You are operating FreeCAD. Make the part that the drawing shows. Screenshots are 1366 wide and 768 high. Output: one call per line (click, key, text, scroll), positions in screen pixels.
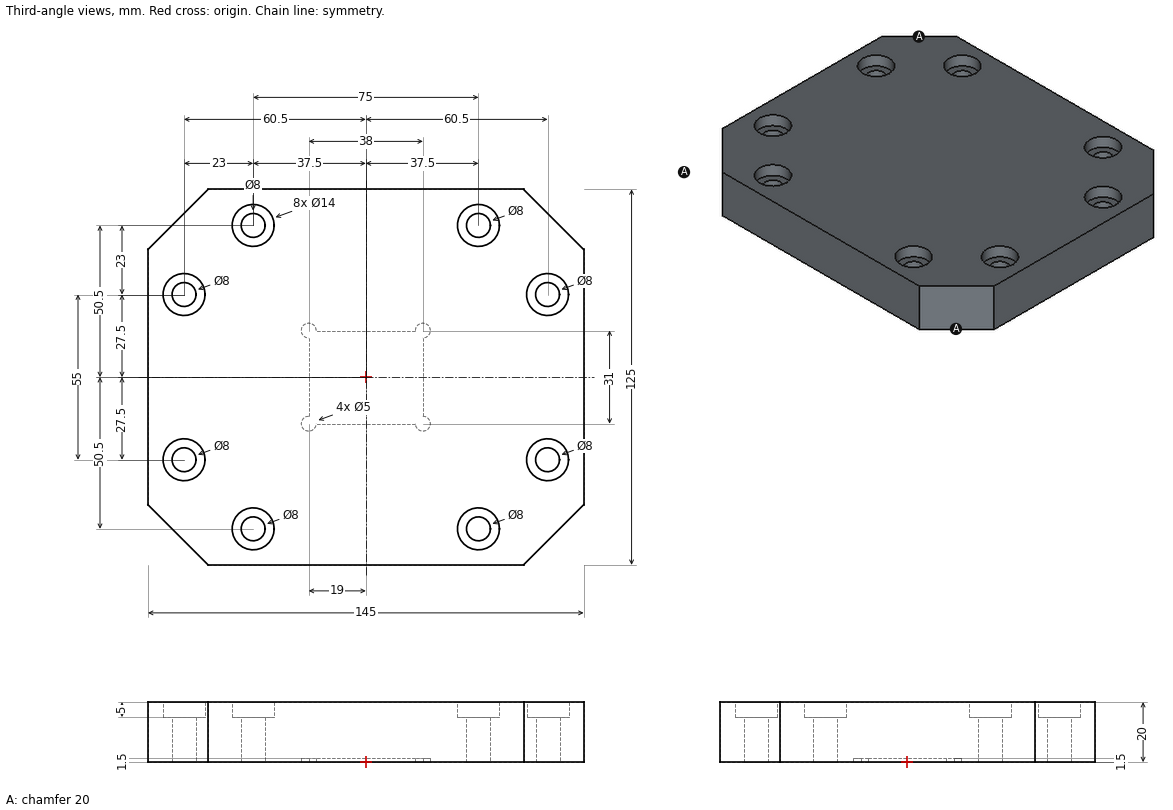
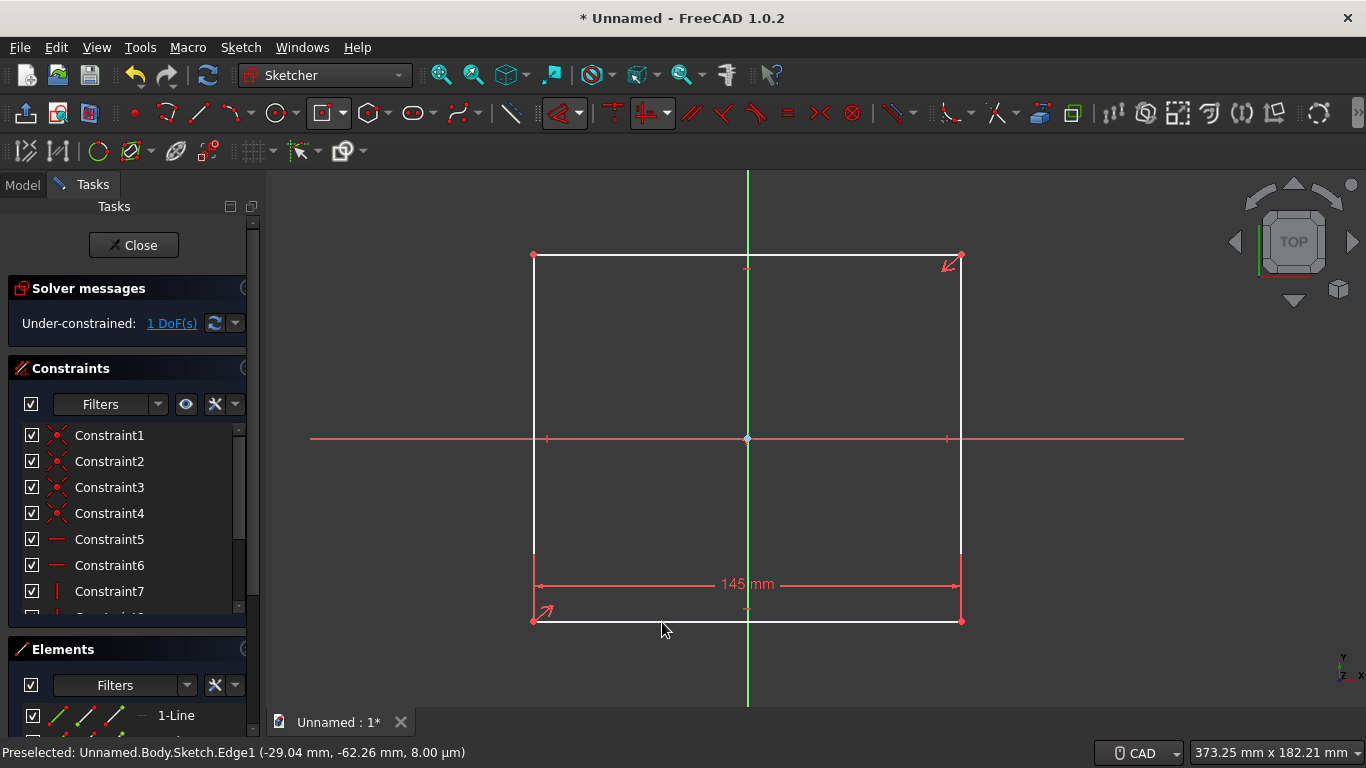
click(961, 512)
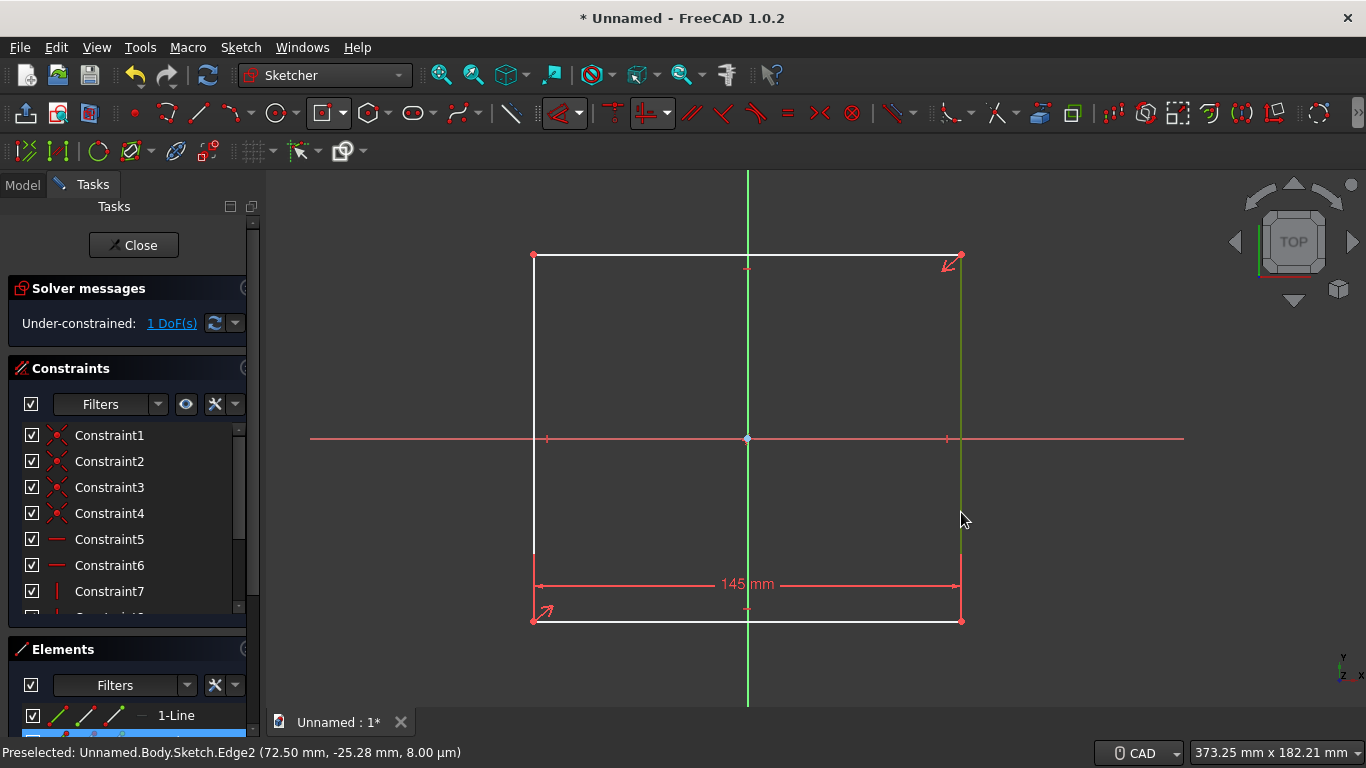
click(582, 114)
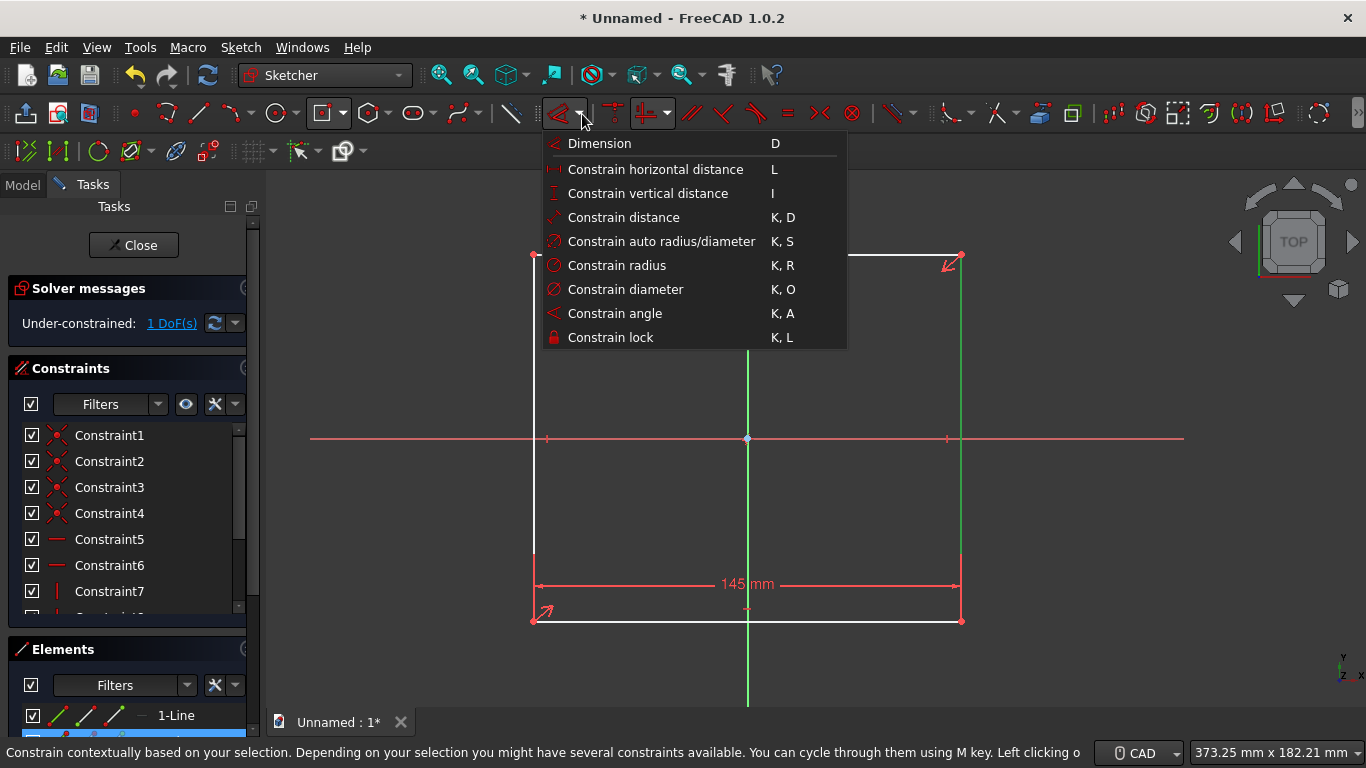
click(695, 193)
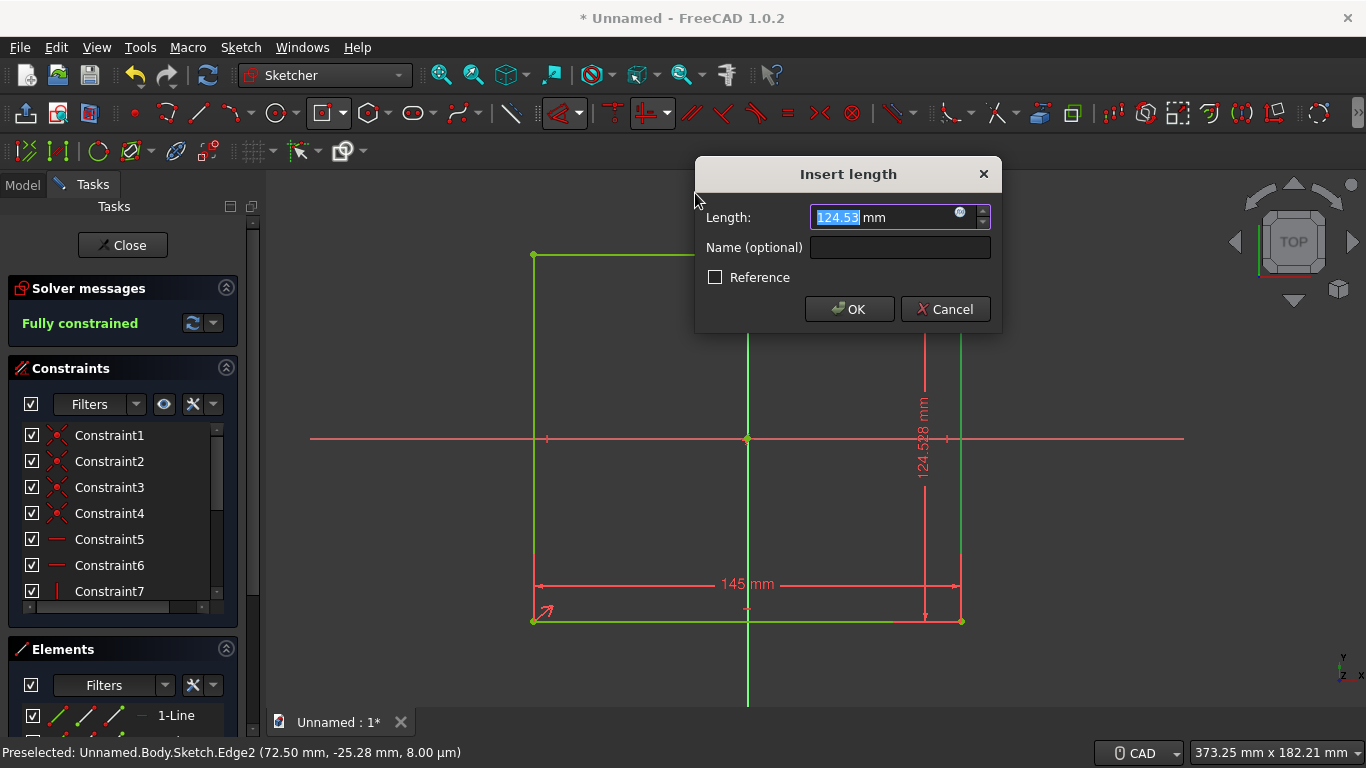
text(125)
key(Return)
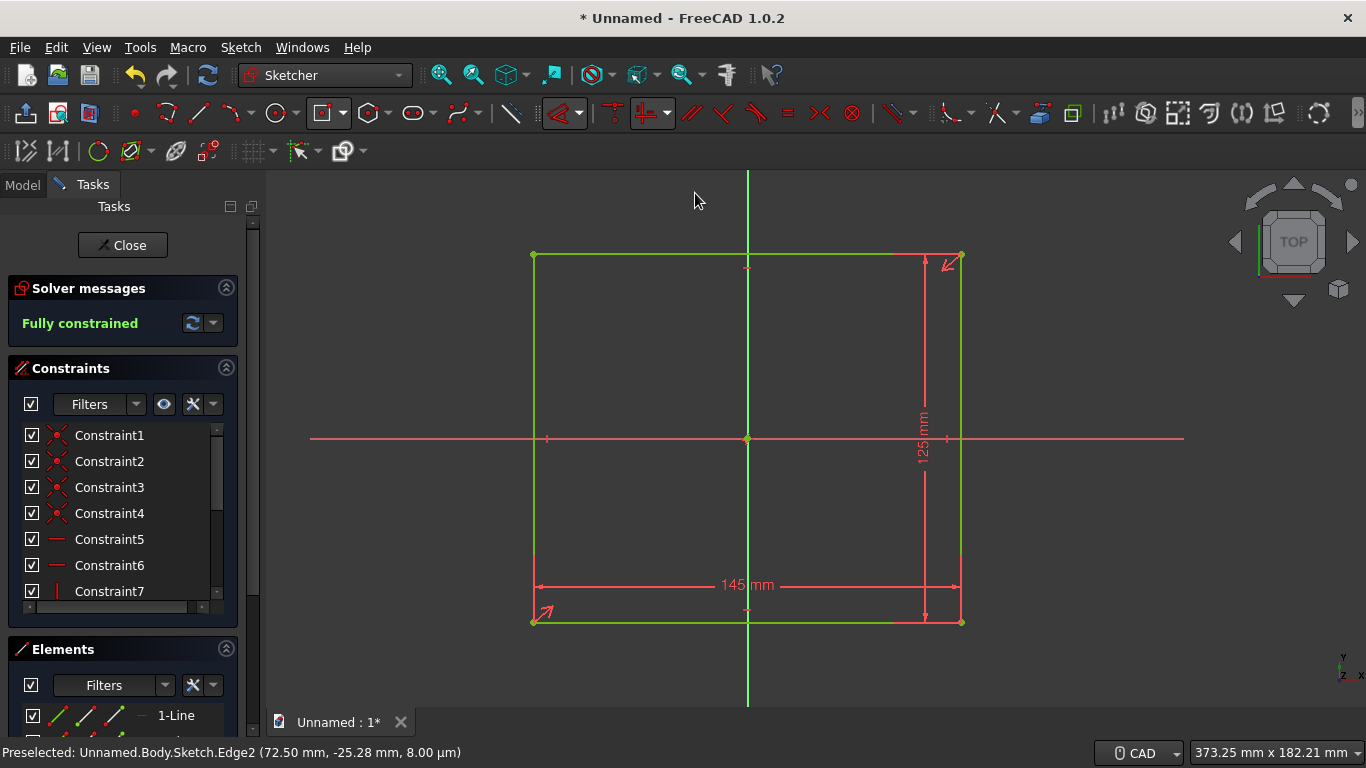
click(123, 245)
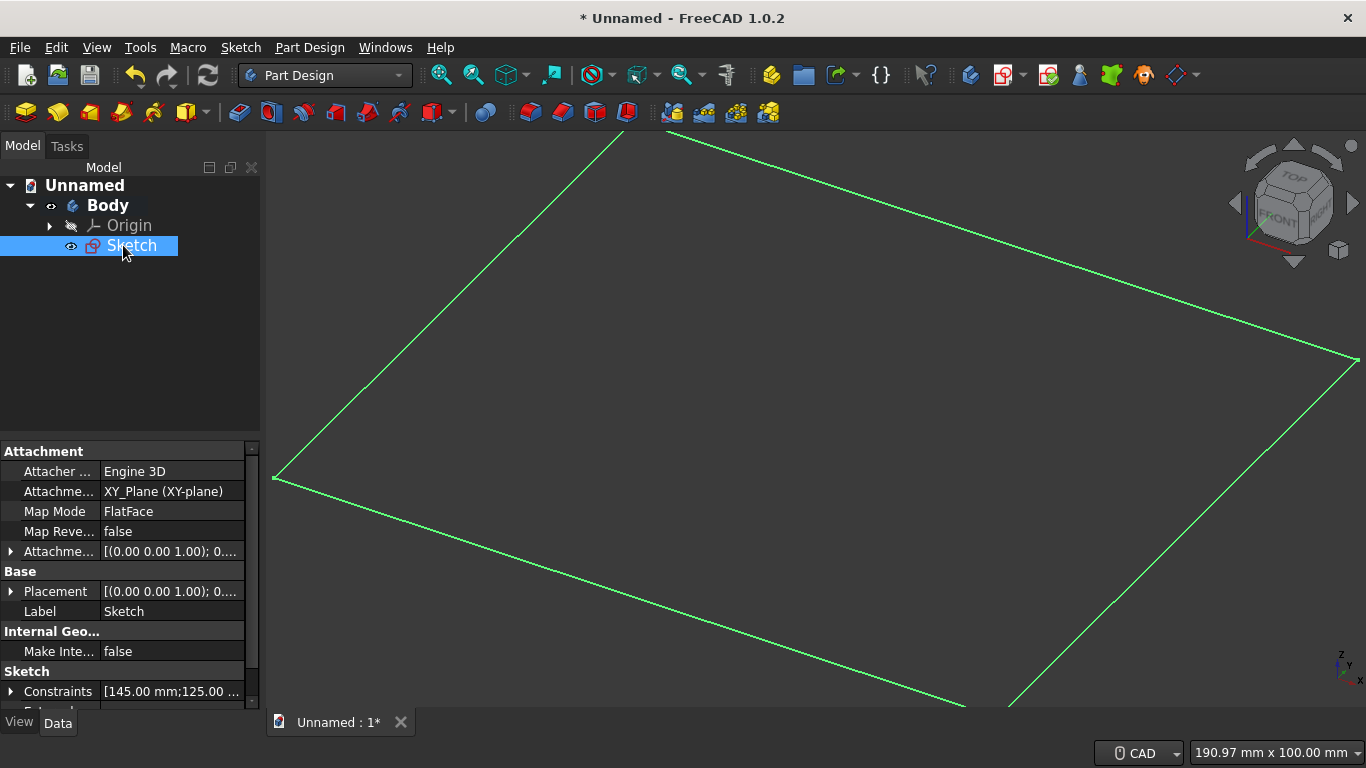
click(26, 112)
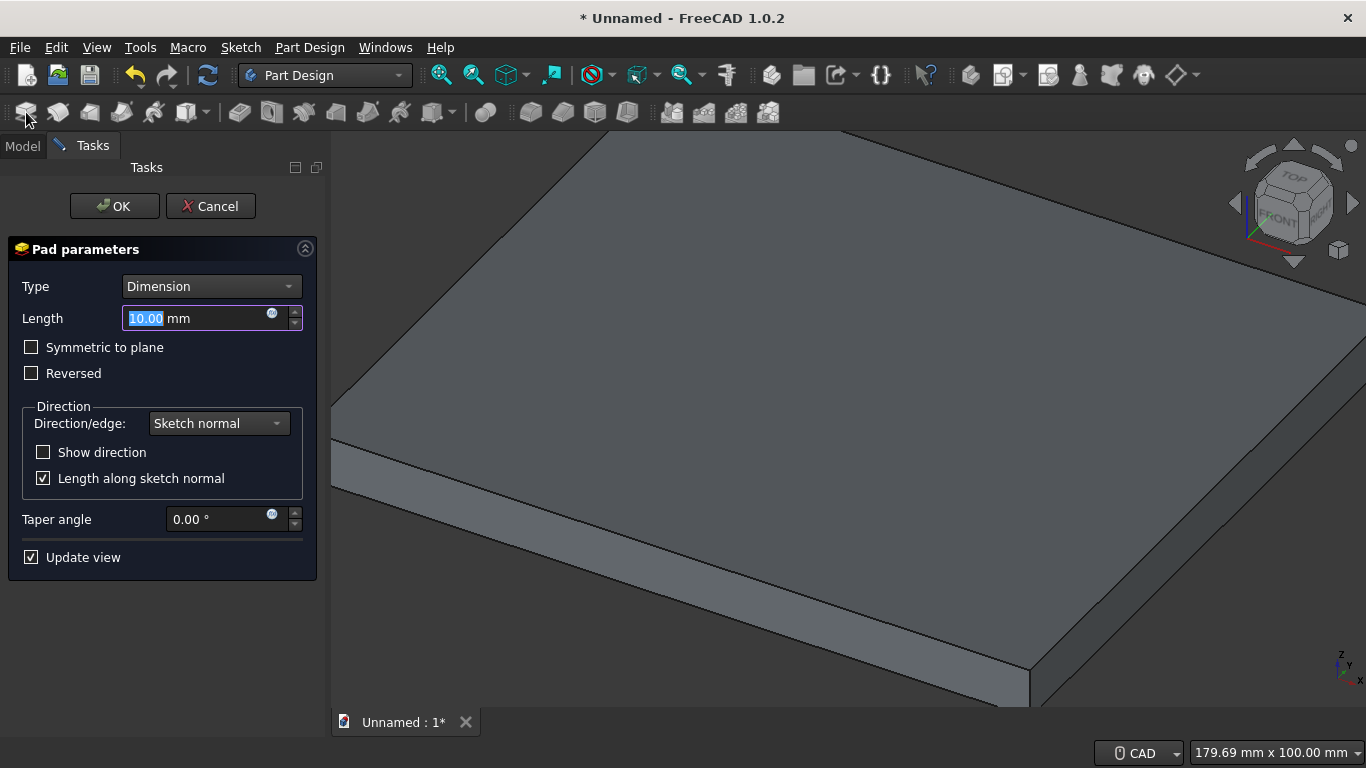
text(20)
key(Tab)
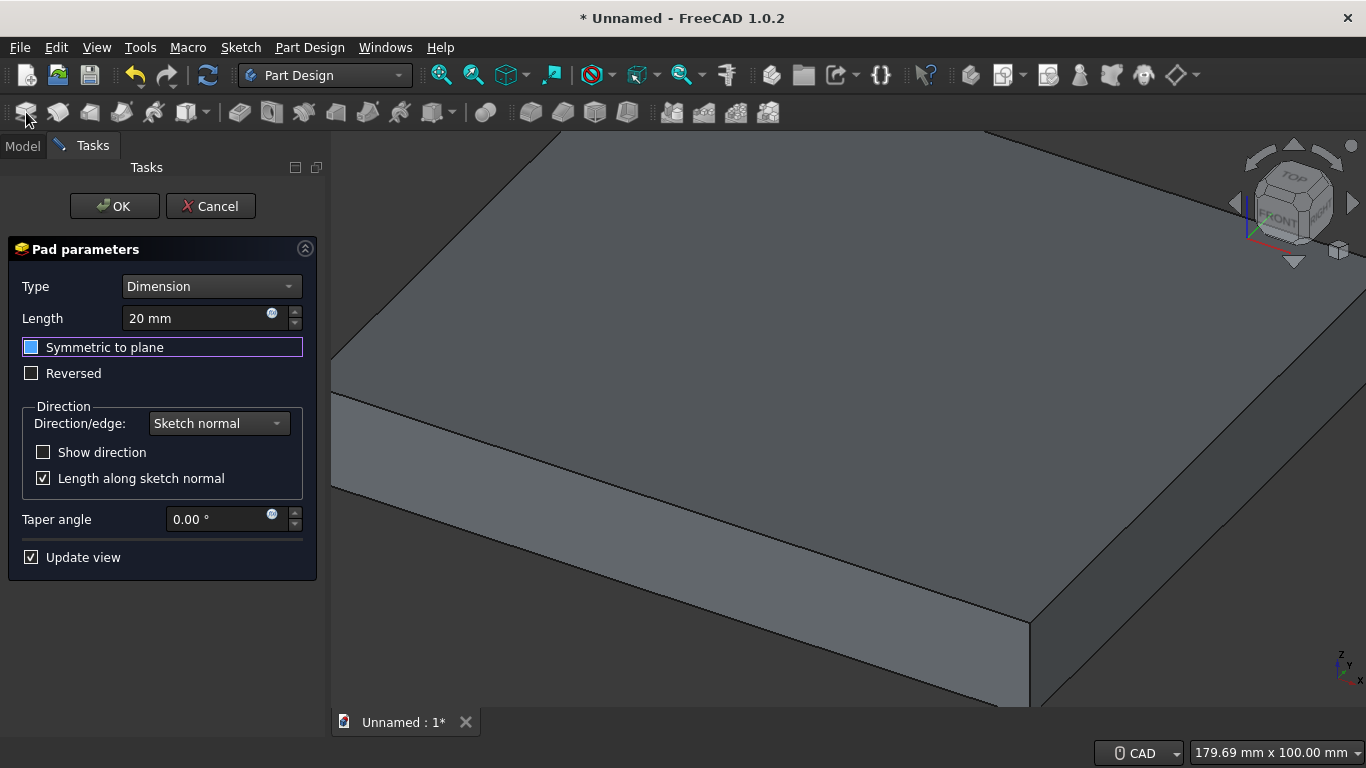
click(115, 206)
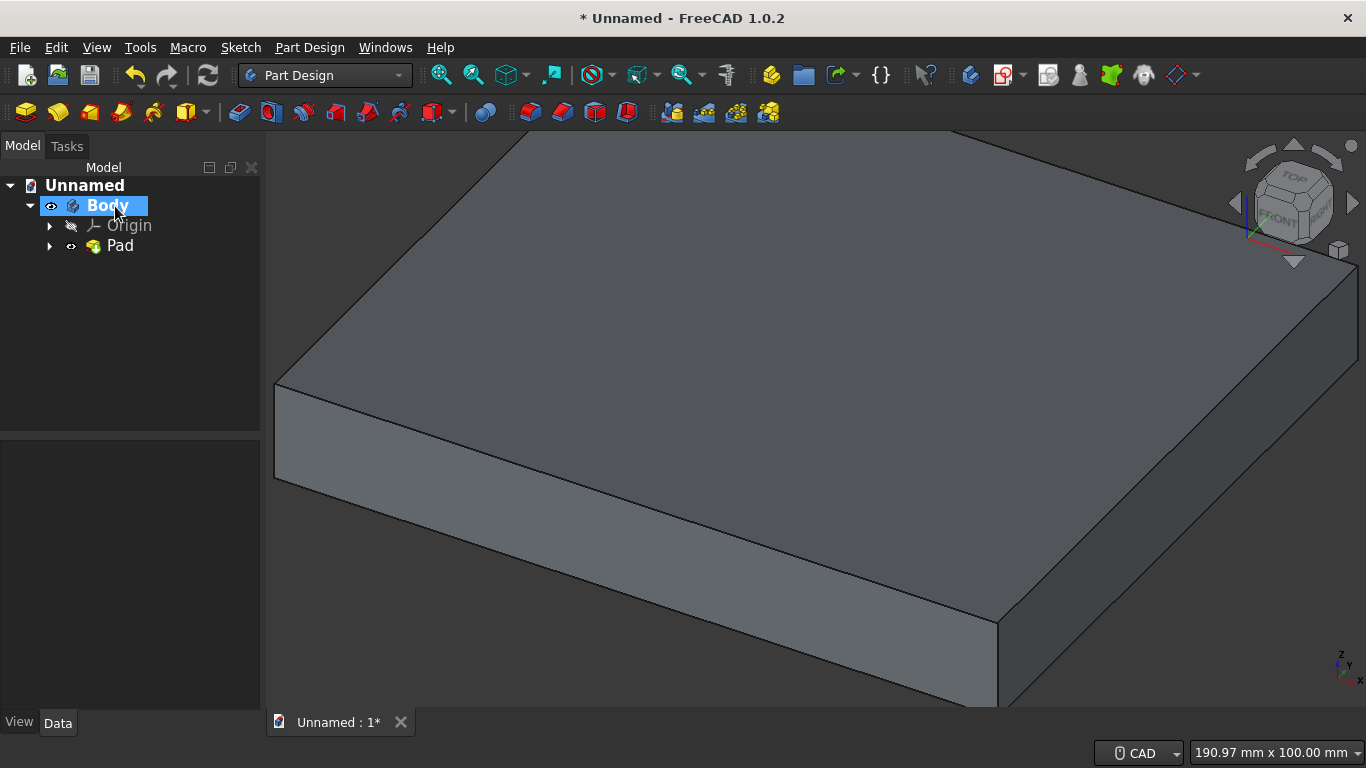
key(v)
key(f)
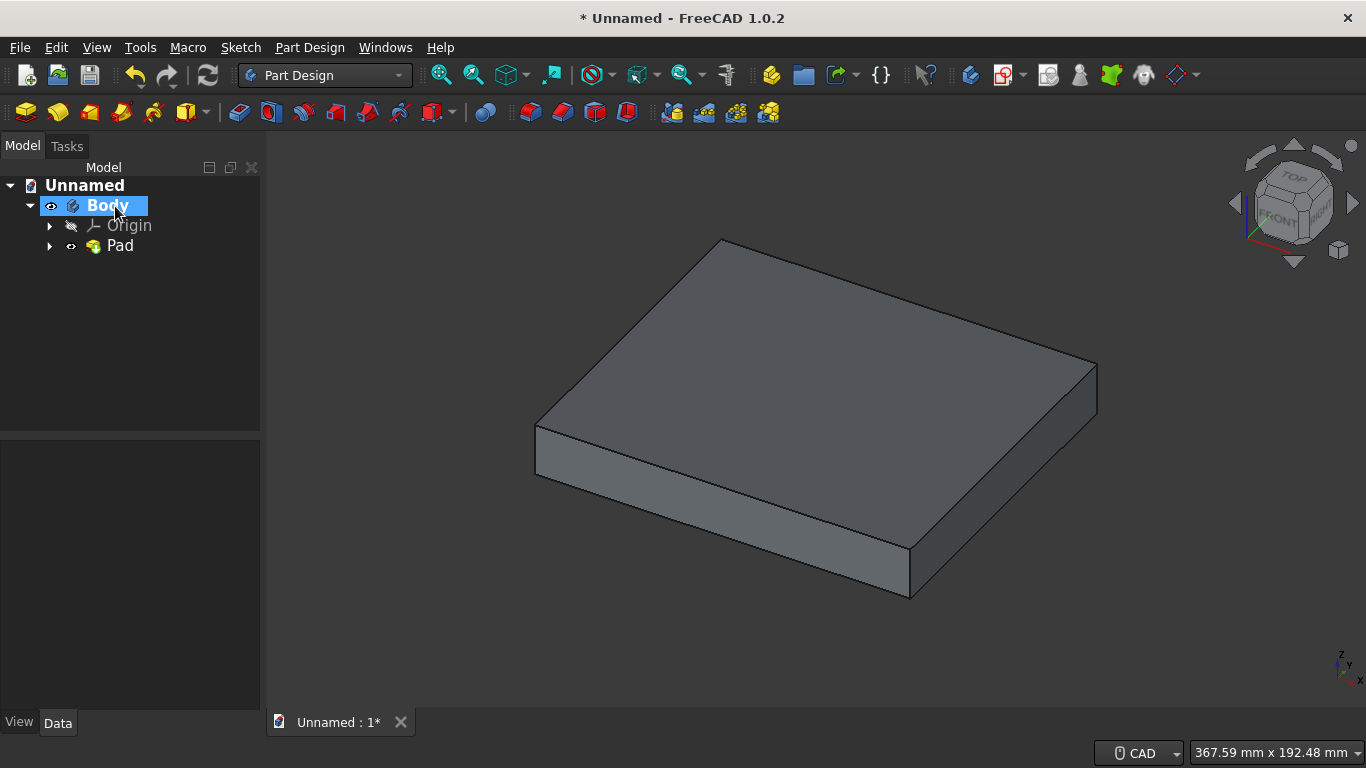
click(910, 573)